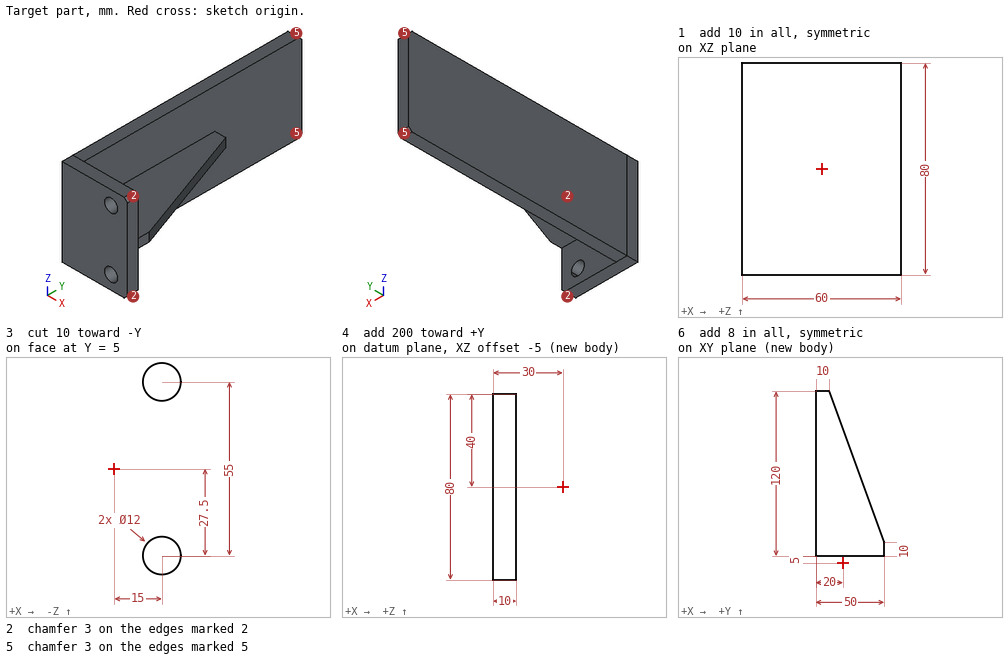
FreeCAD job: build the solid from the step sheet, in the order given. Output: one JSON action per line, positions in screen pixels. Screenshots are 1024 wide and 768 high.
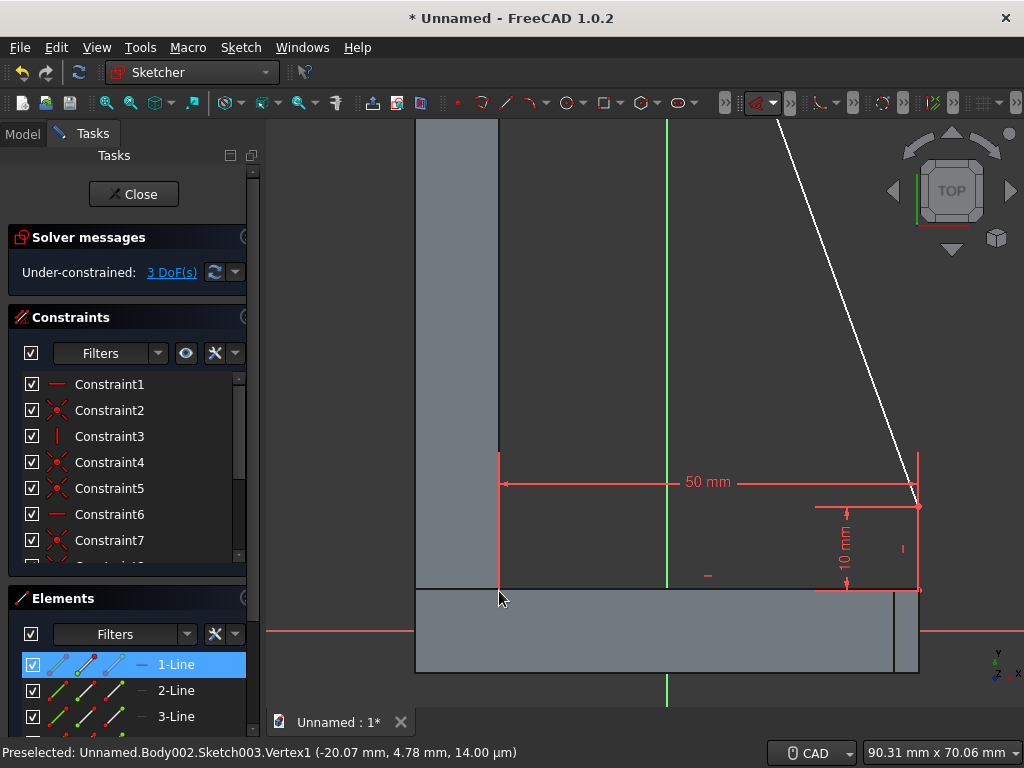
{"action": "left_click", "coordinate": [776, 104]}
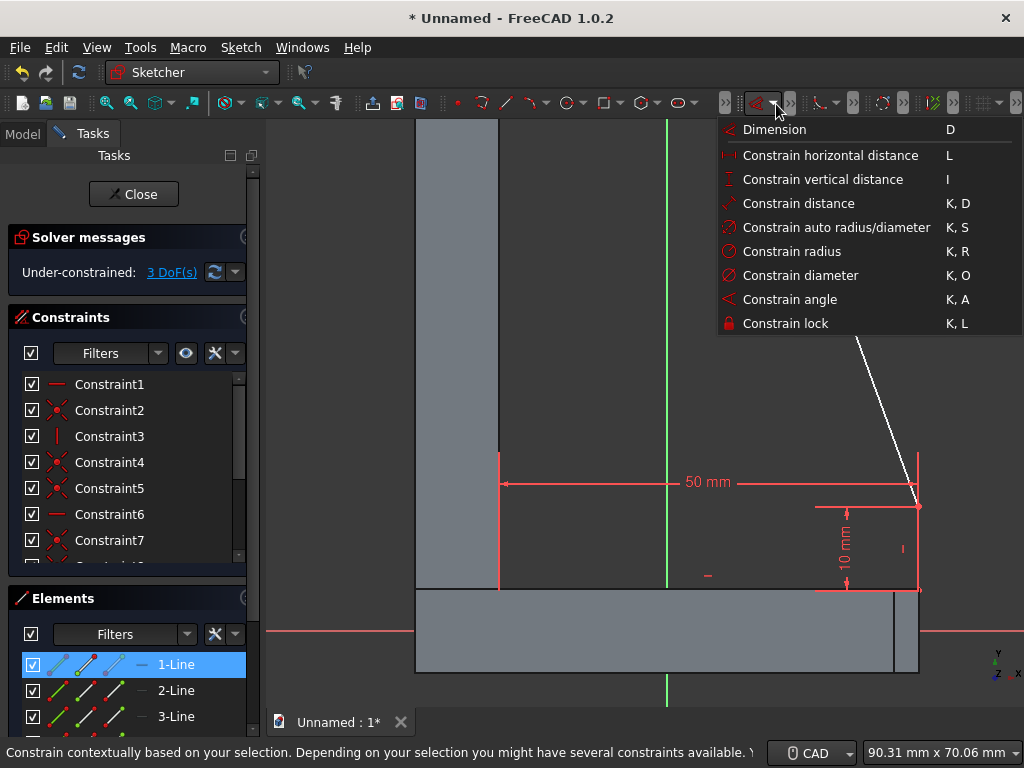
{"action": "left_click", "coordinate": [870, 179]}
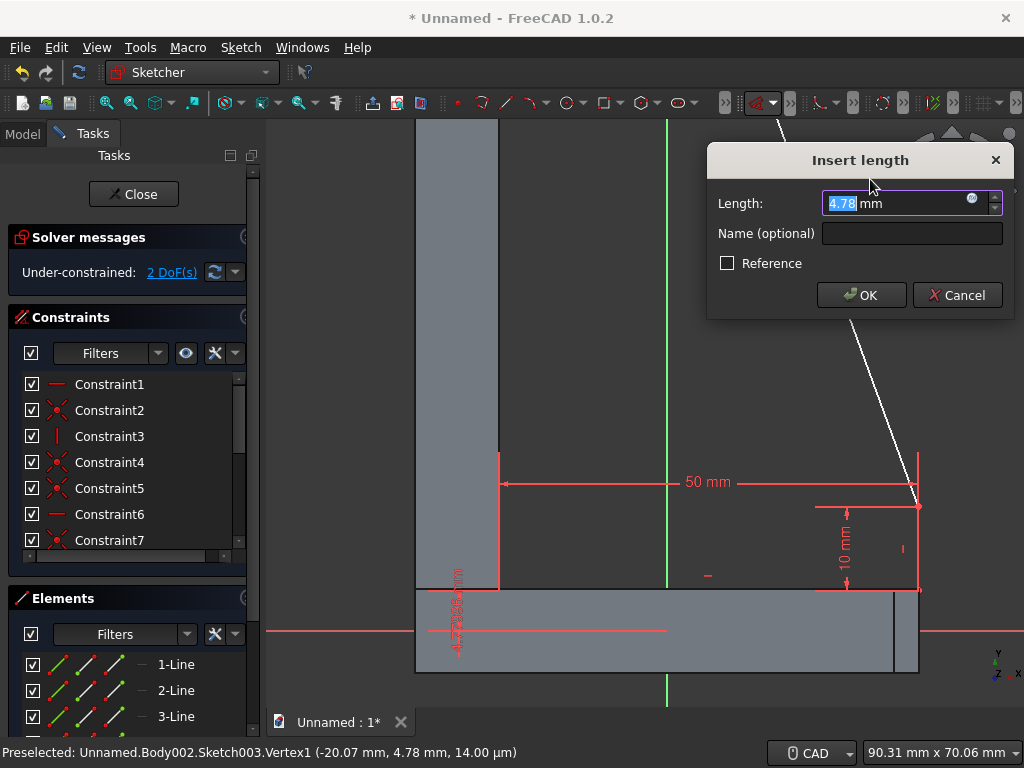
{"action": "type", "text": "5"}
{"action": "key", "text": "Return"}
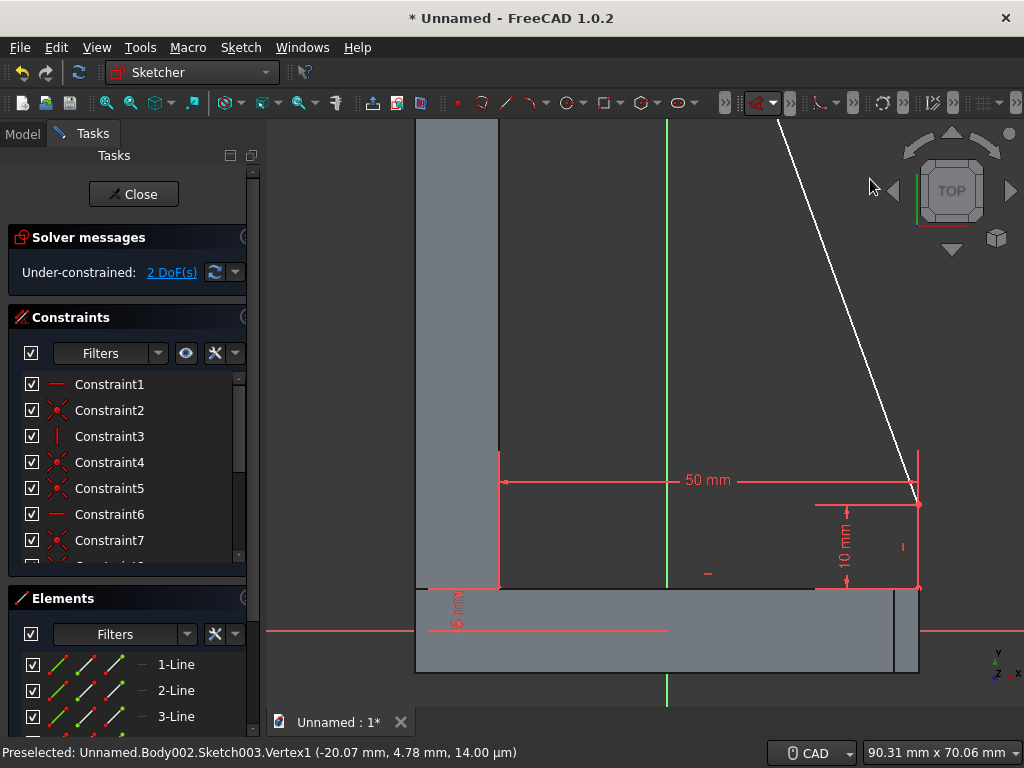
{"action": "left_click", "coordinate": [499, 287]}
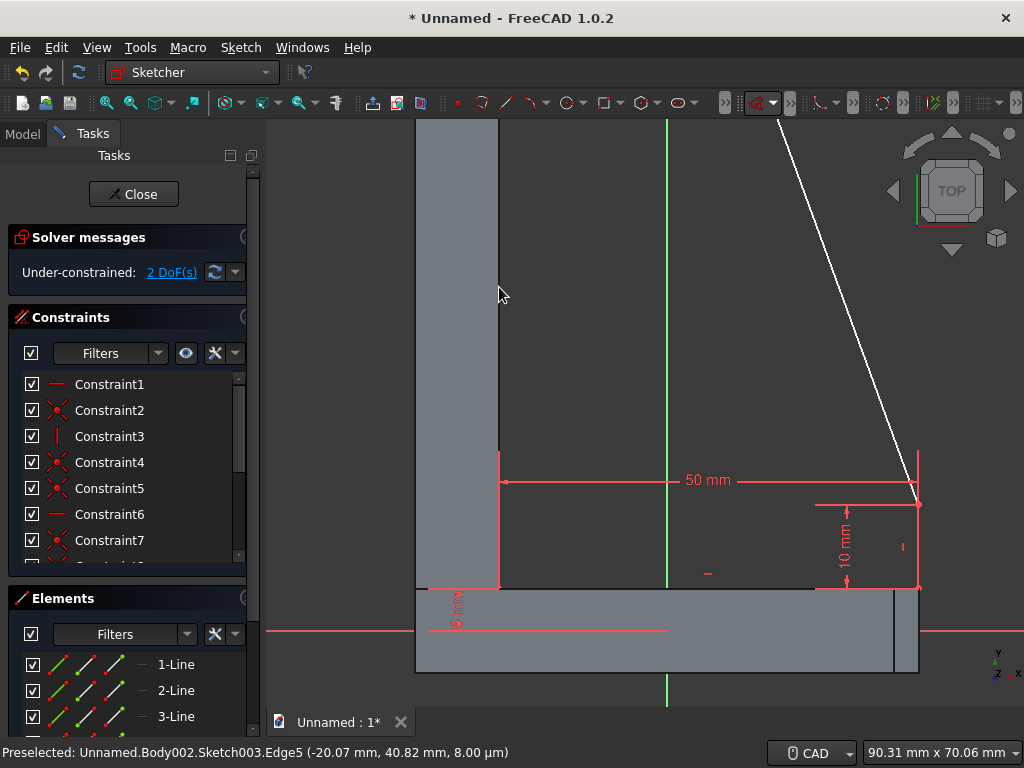
{"action": "left_click", "coordinate": [776, 104]}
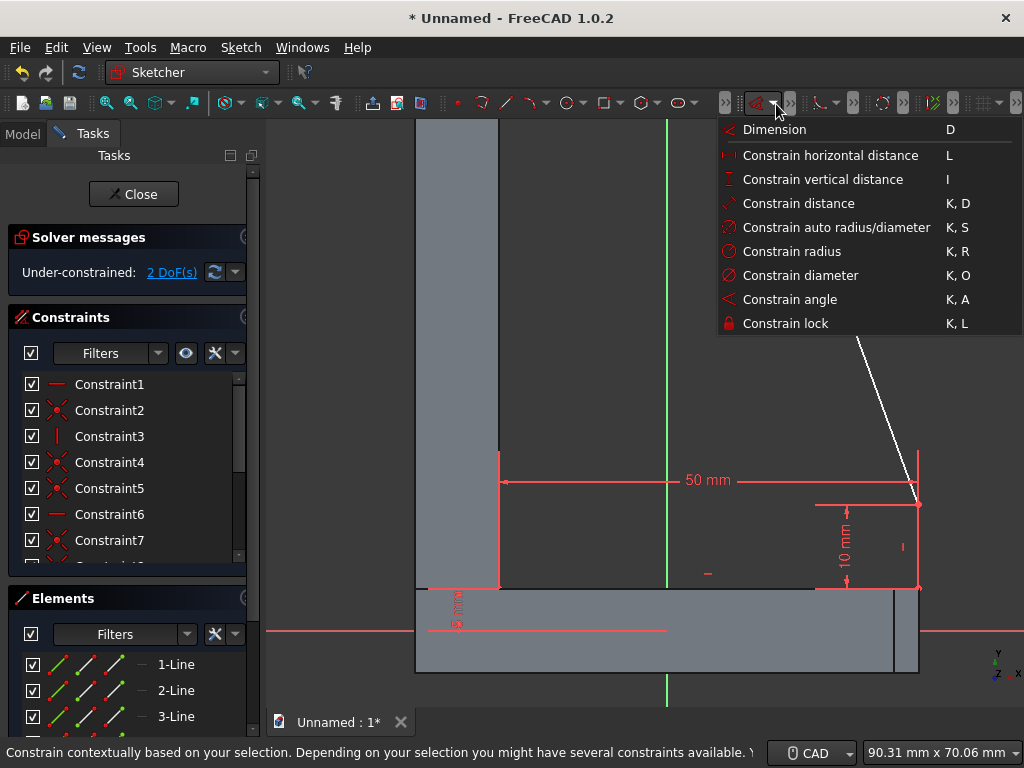
{"action": "left_click", "coordinate": [870, 179]}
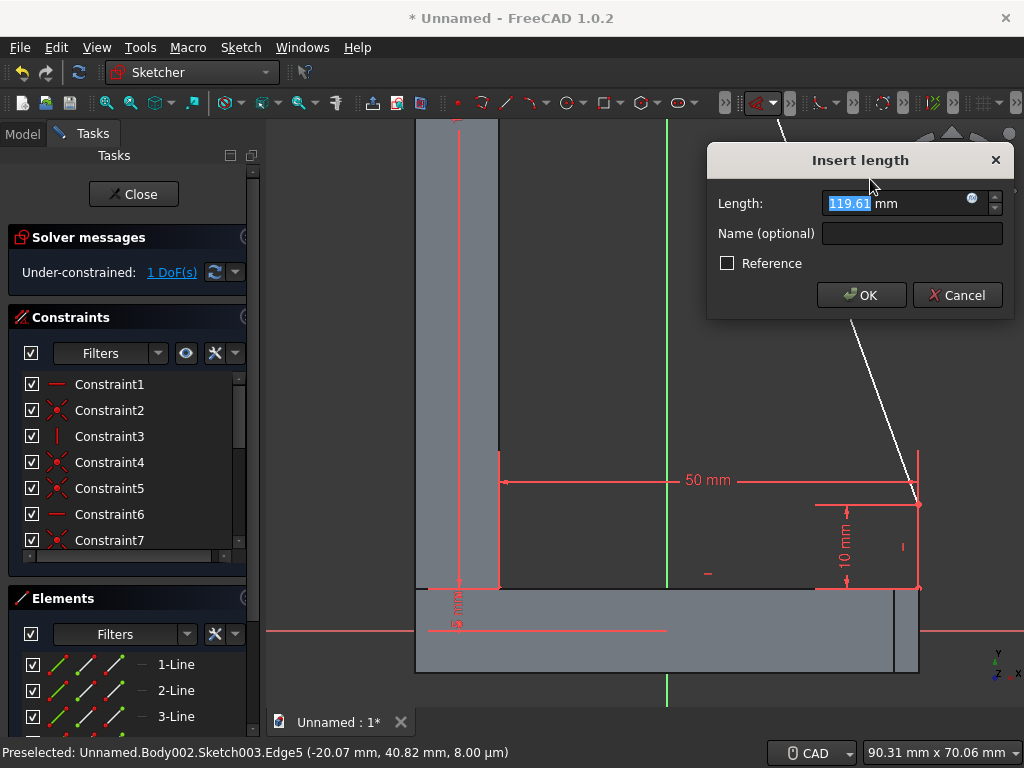
{"action": "type", "text": "120"}
{"action": "key", "text": "Return"}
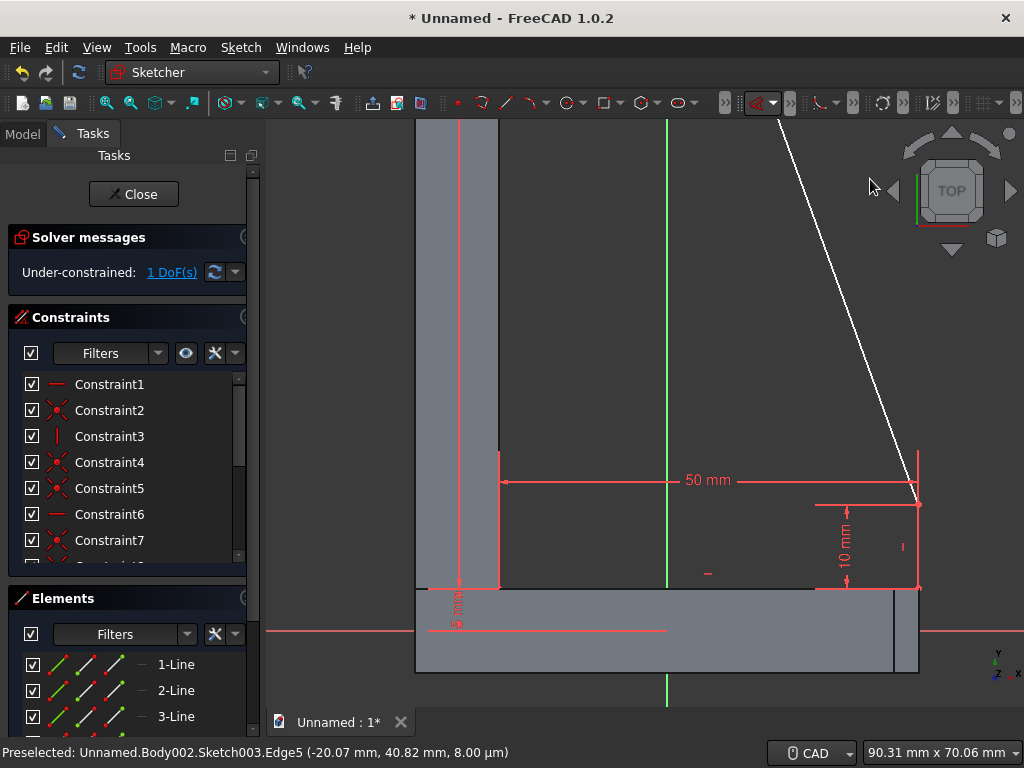
{"action": "left_click", "coordinate": [499, 589]}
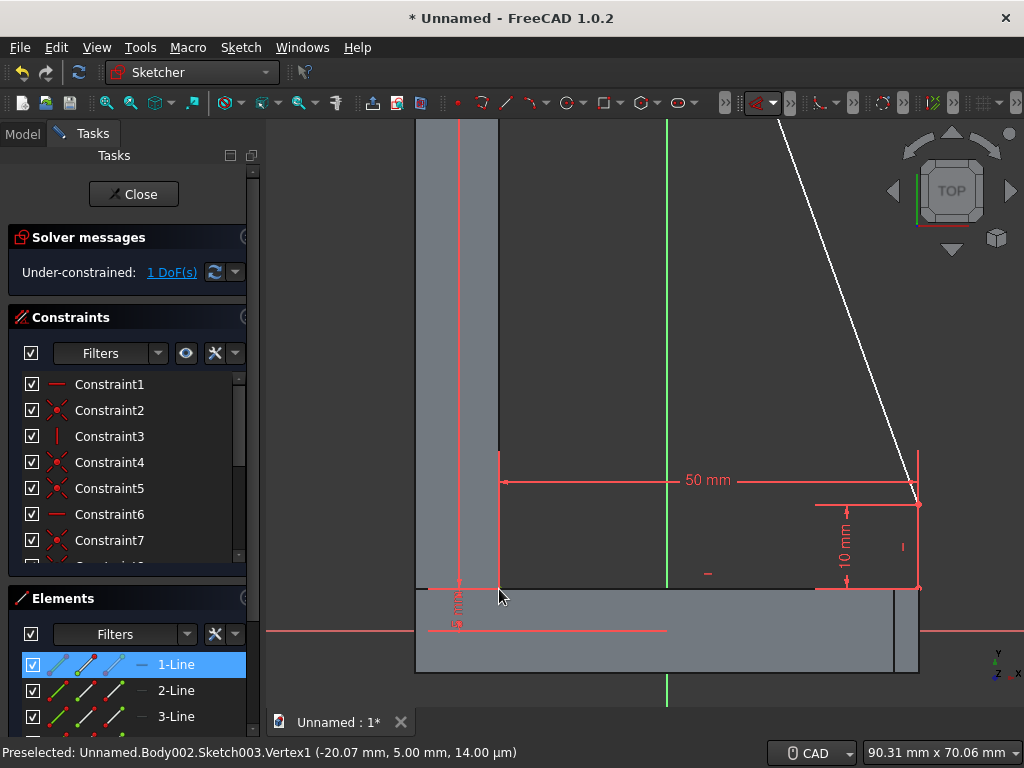
{"action": "left_click", "coordinate": [776, 104]}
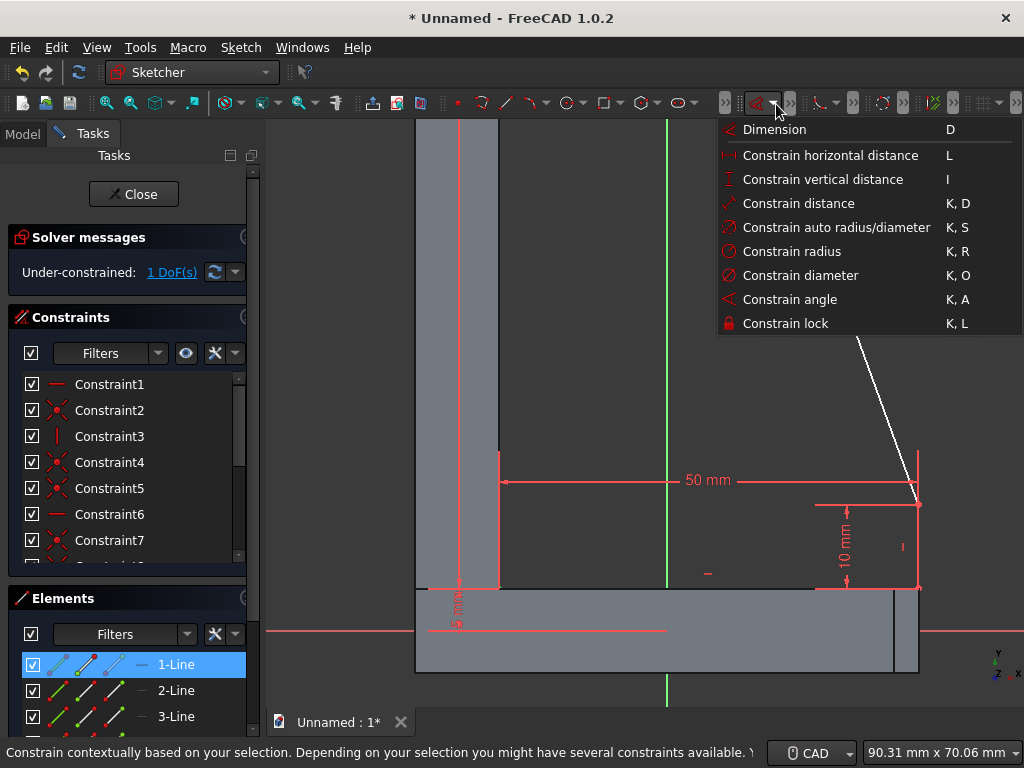
{"action": "left_click", "coordinate": [870, 155]}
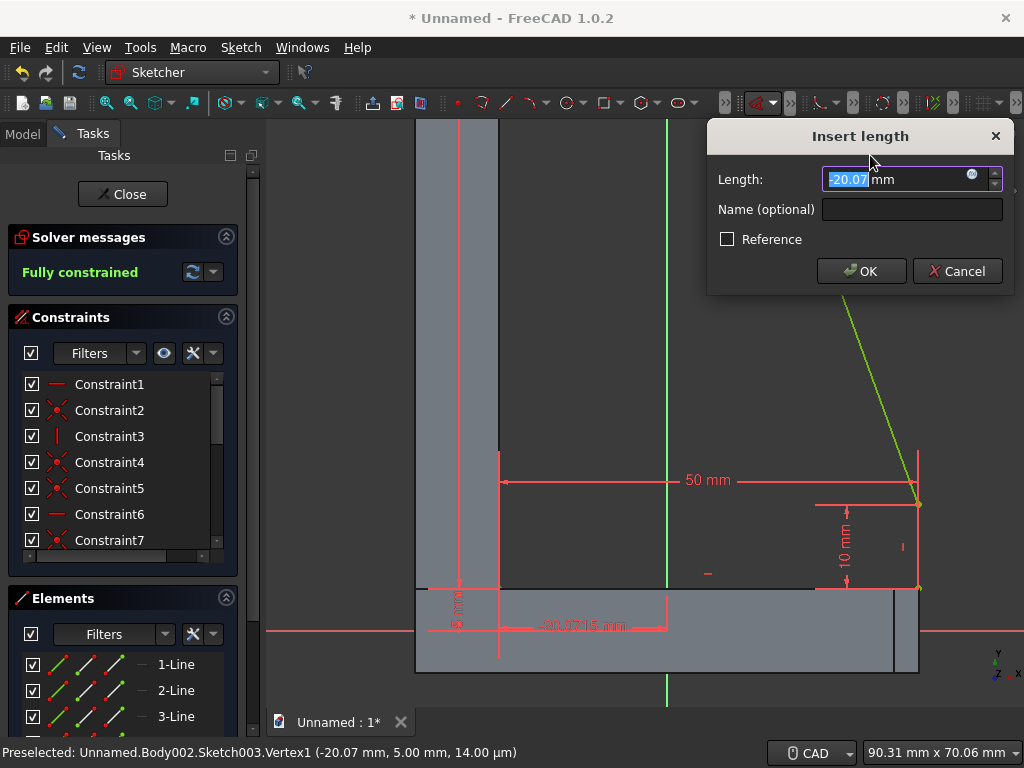
{"action": "type", "text": "-20"}
{"action": "key", "text": "Return"}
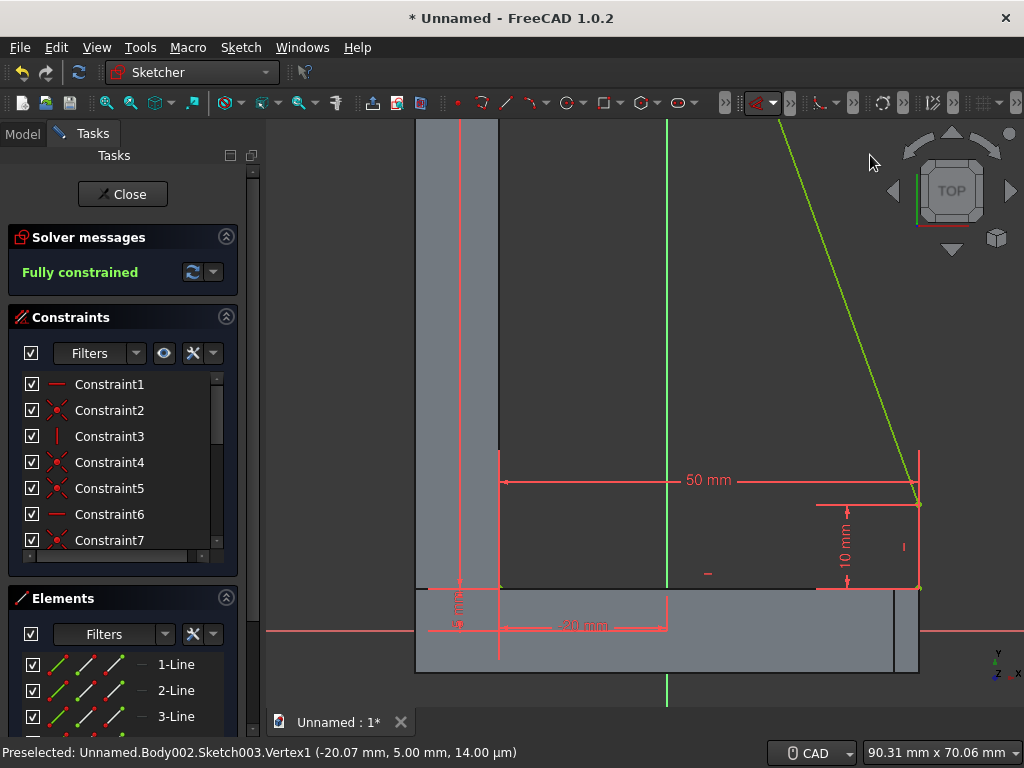
{"action": "left_click", "coordinate": [123, 194]}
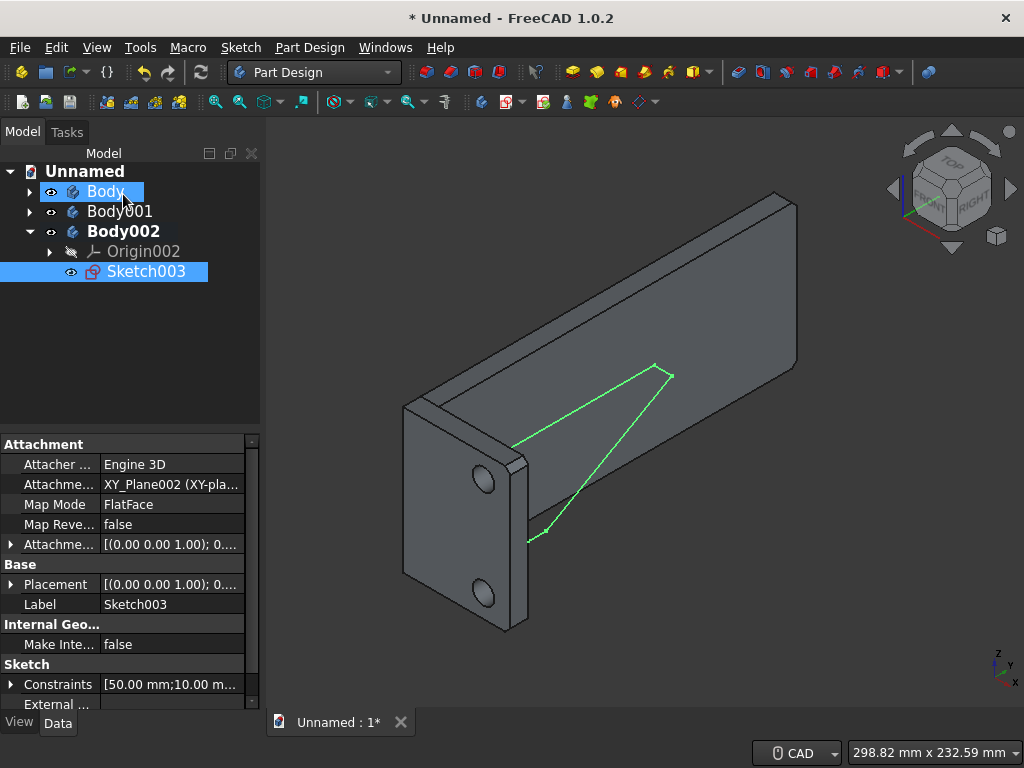
{"action": "left_click", "coordinate": [574, 72]}